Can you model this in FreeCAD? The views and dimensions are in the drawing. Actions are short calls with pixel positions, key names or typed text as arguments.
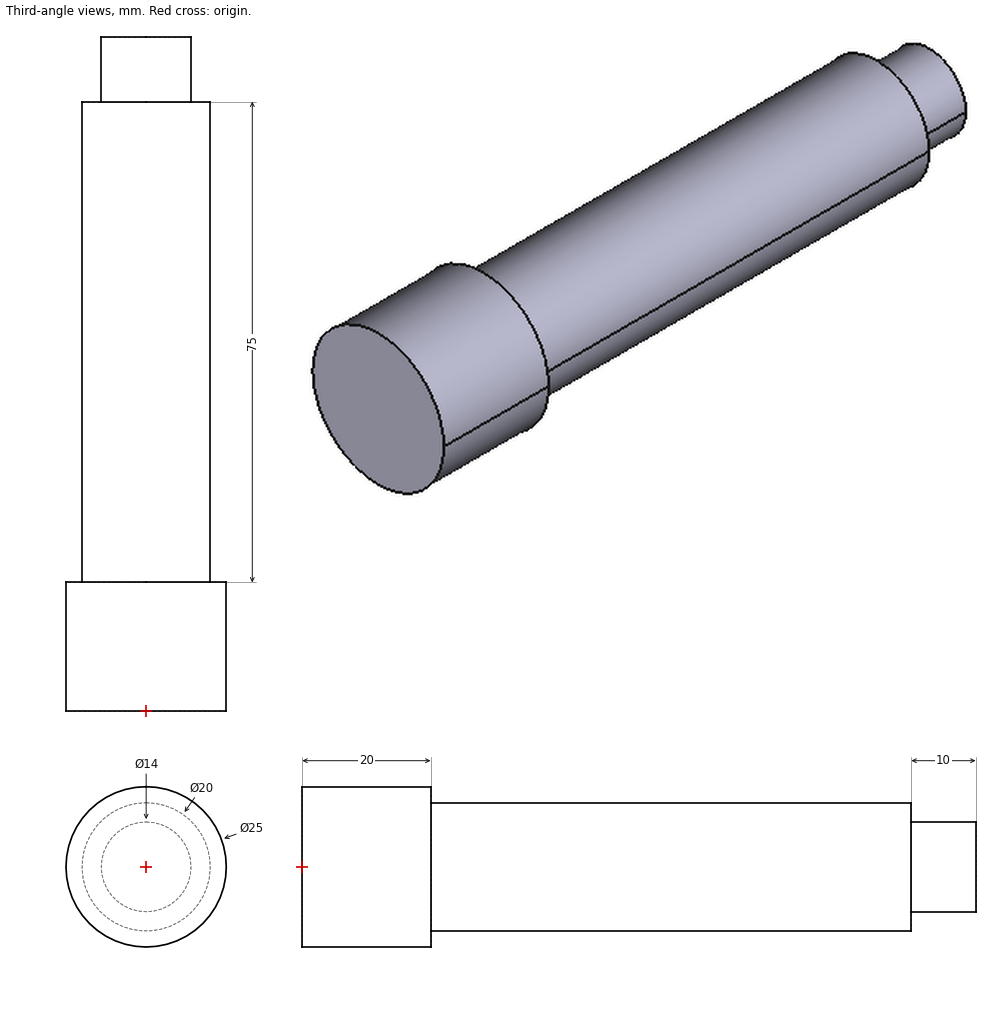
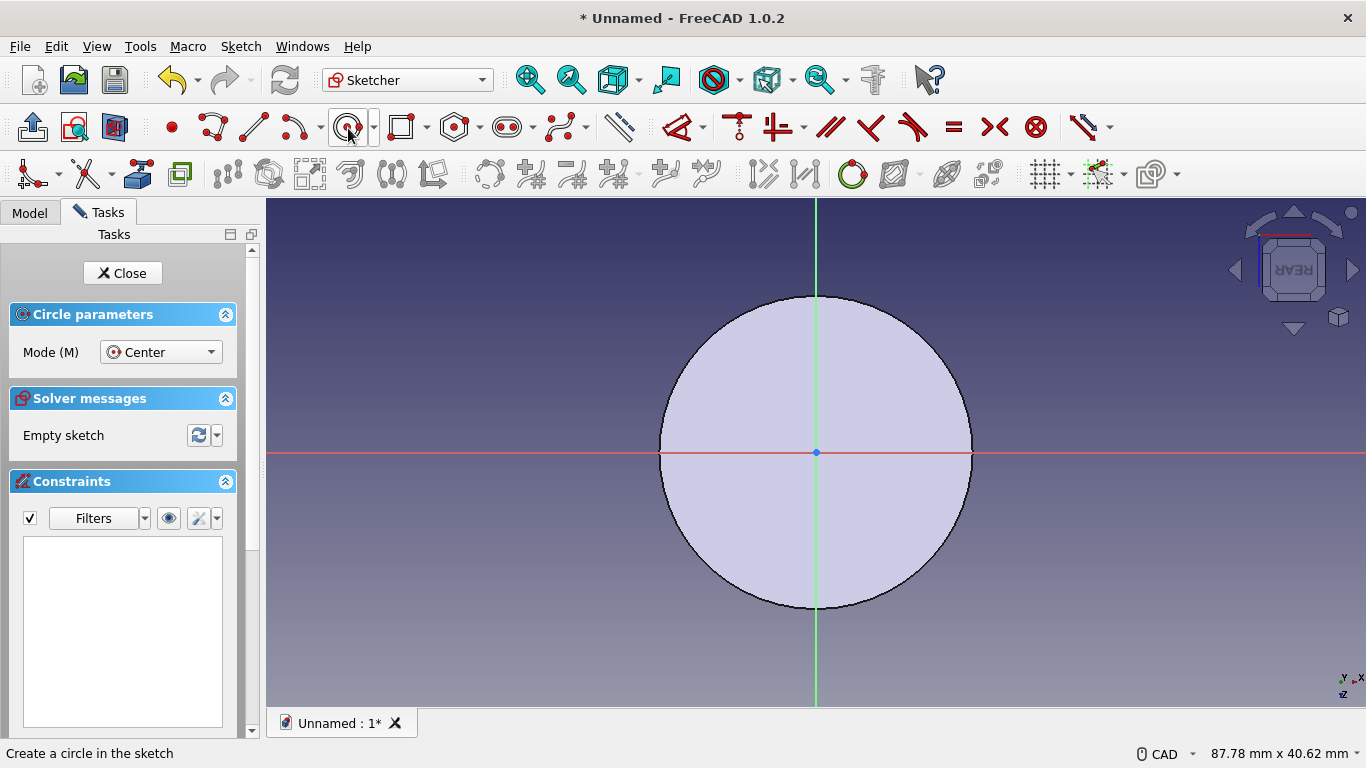
click(816, 453)
move(905, 364)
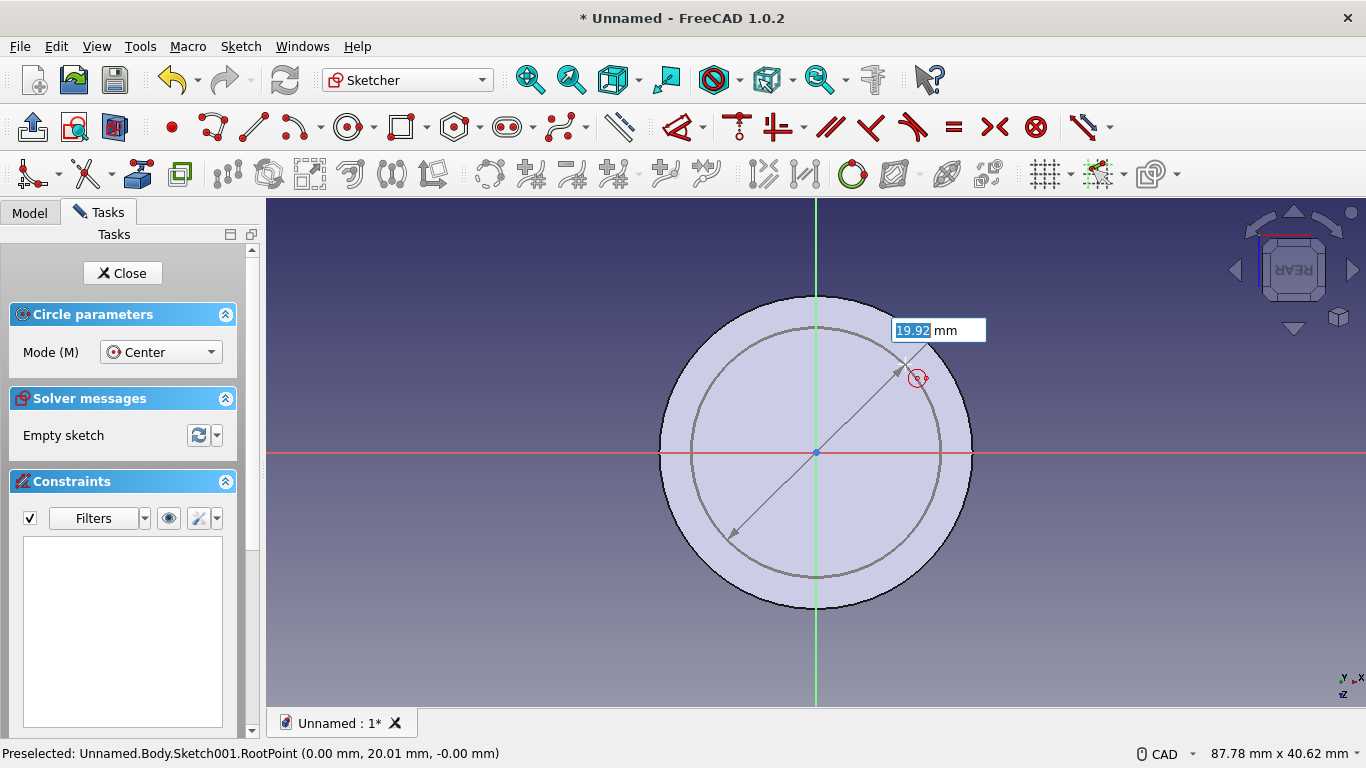
text(20)
key(Return)
key(Escape)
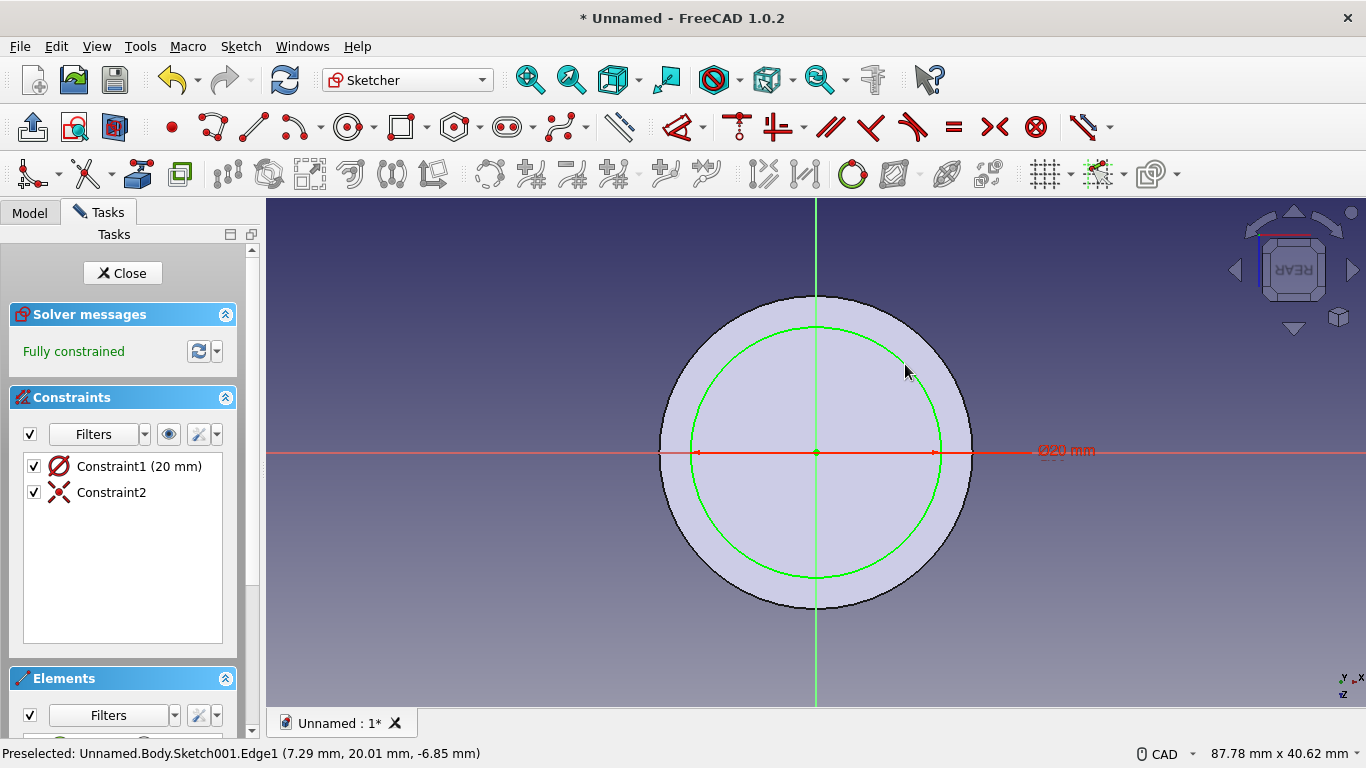
click(123, 273)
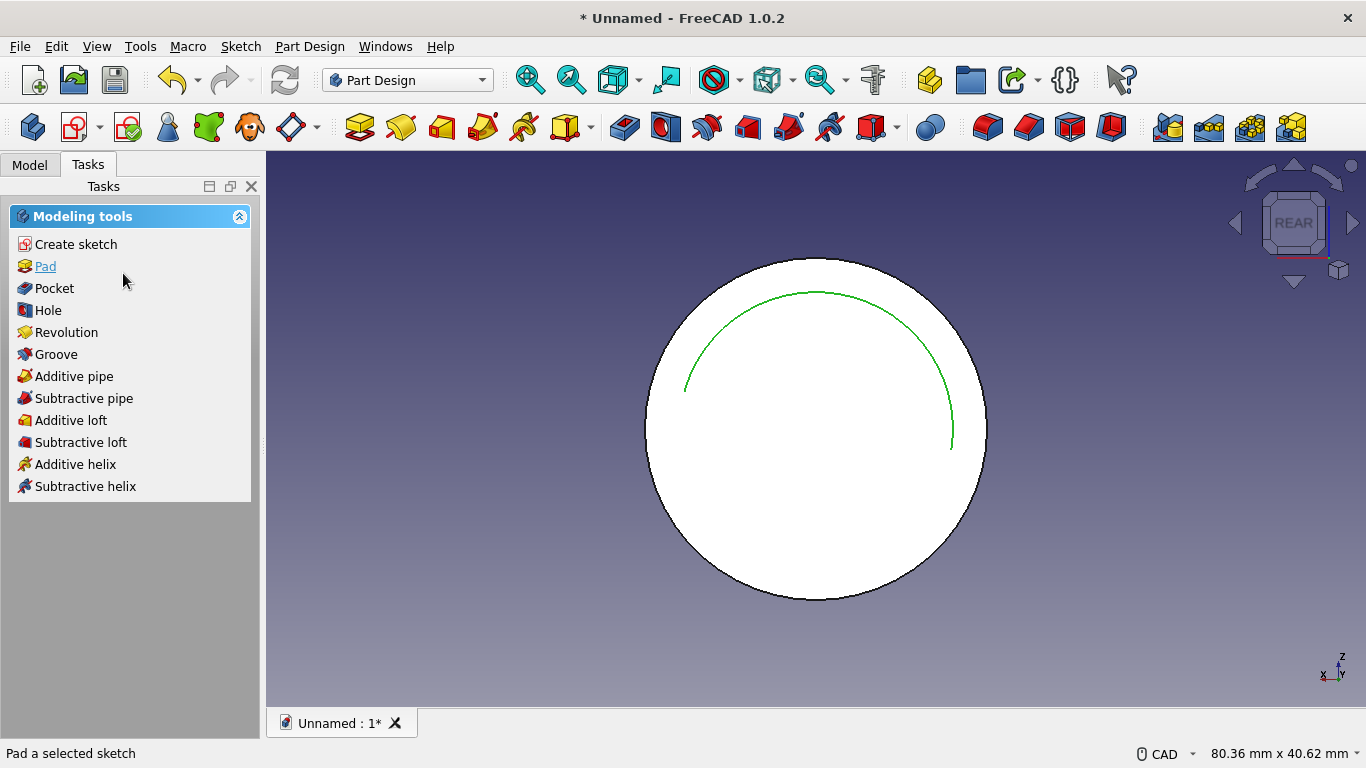
click(360, 128)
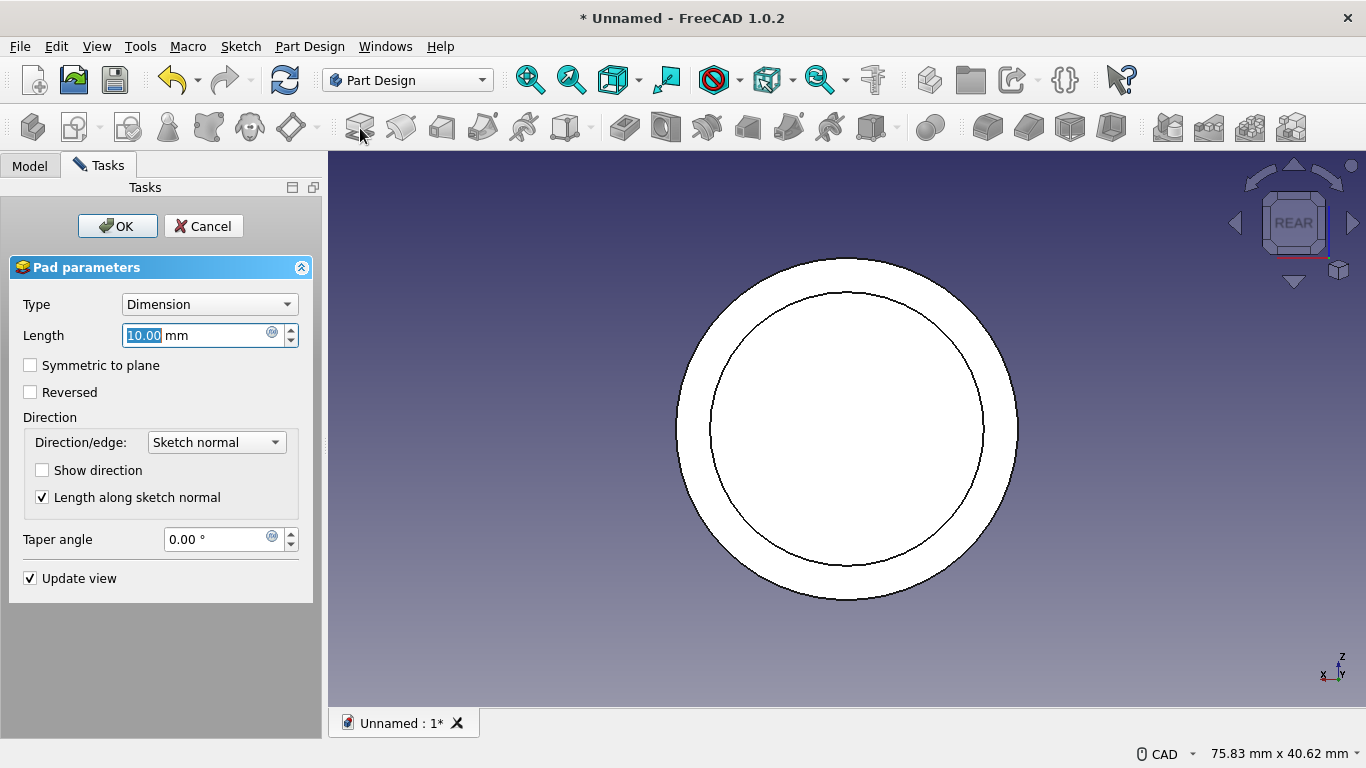
text(75)
key(Tab)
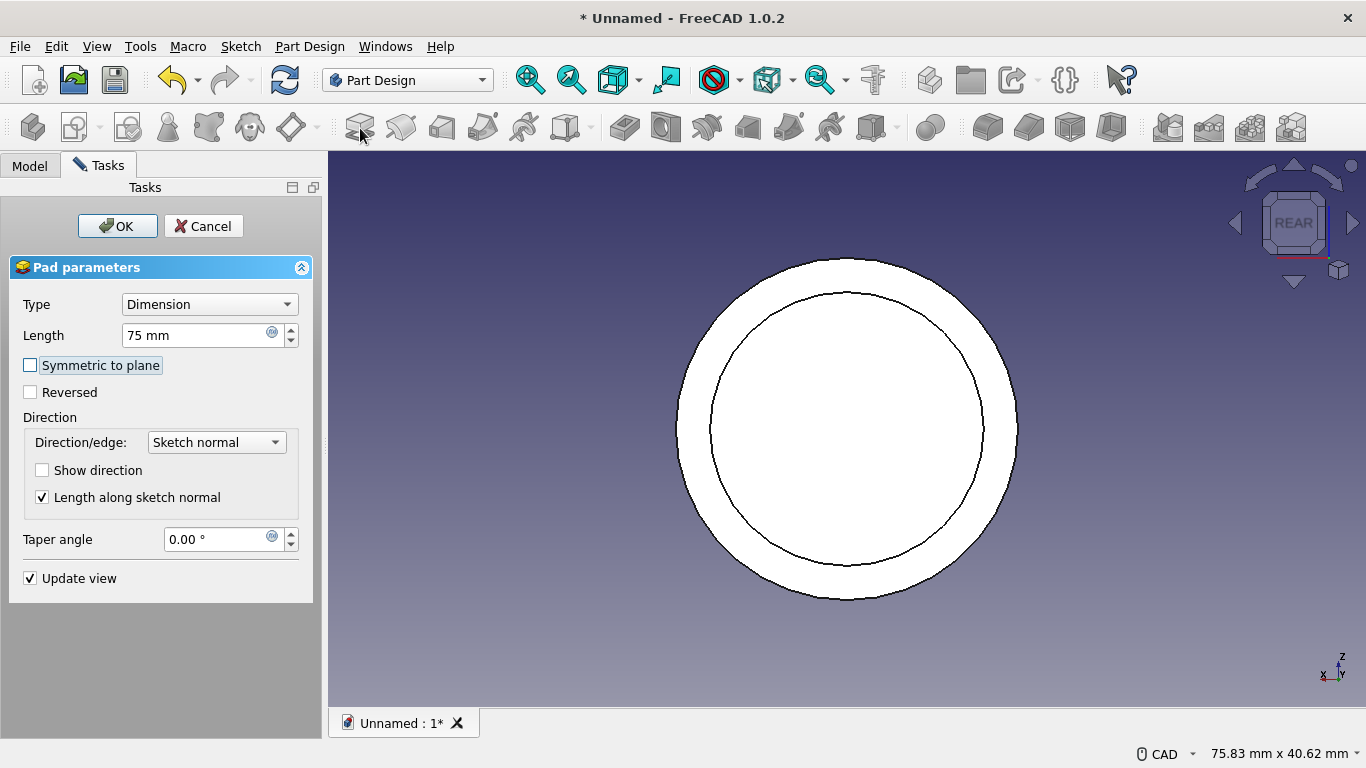
click(118, 226)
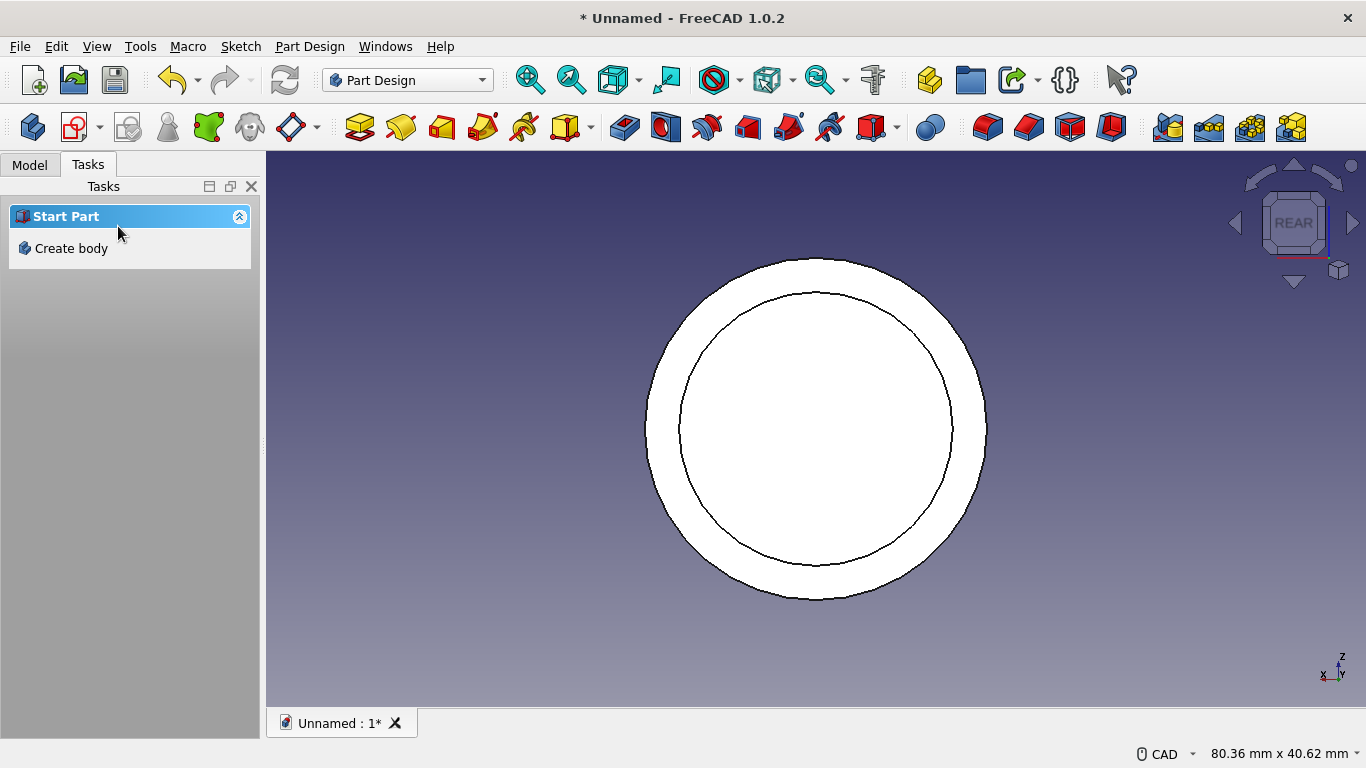
click(816, 428)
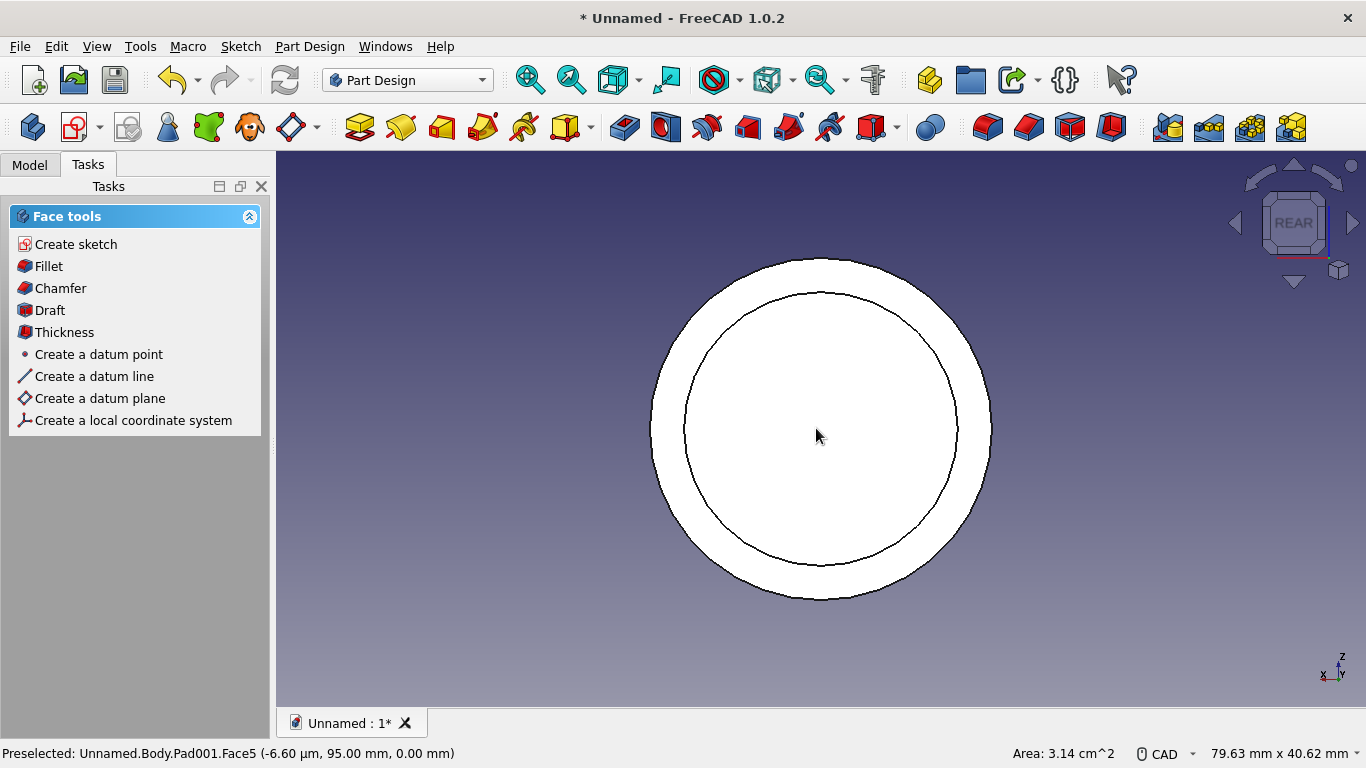
click(74, 128)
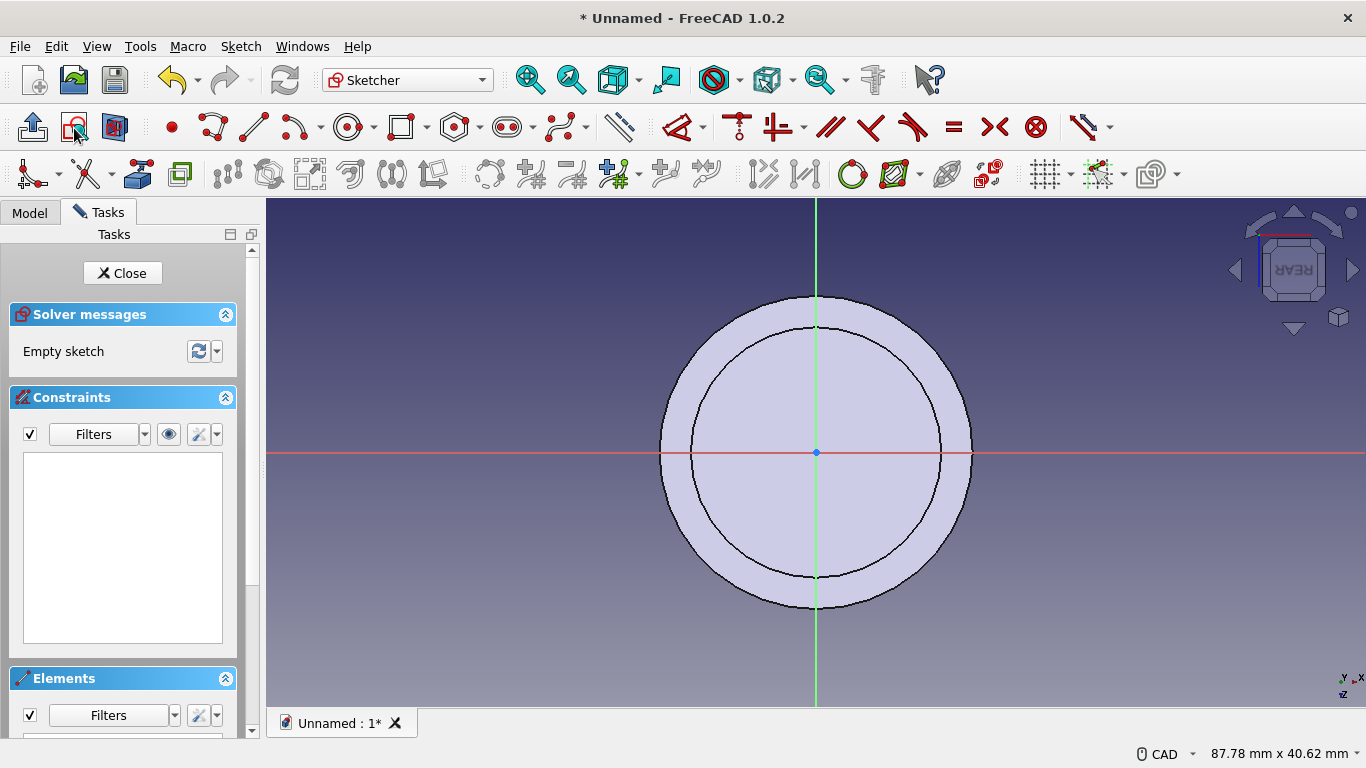
scroll(900, 452, up, 3)